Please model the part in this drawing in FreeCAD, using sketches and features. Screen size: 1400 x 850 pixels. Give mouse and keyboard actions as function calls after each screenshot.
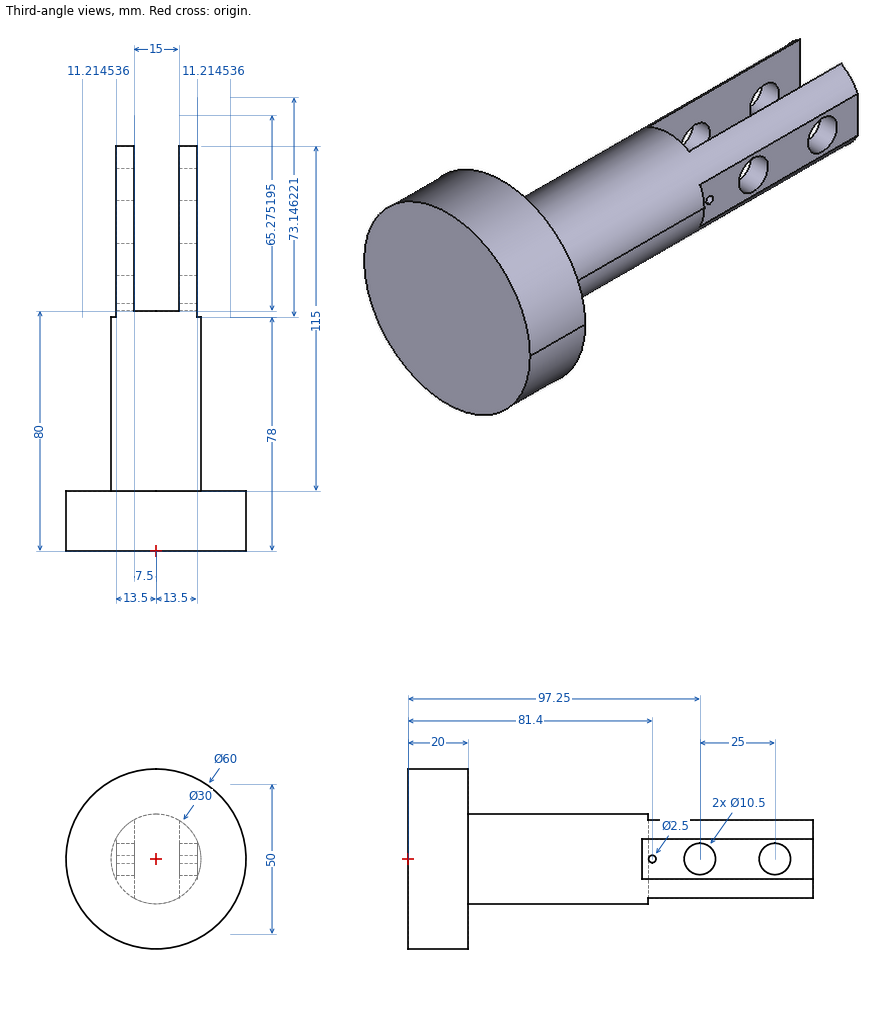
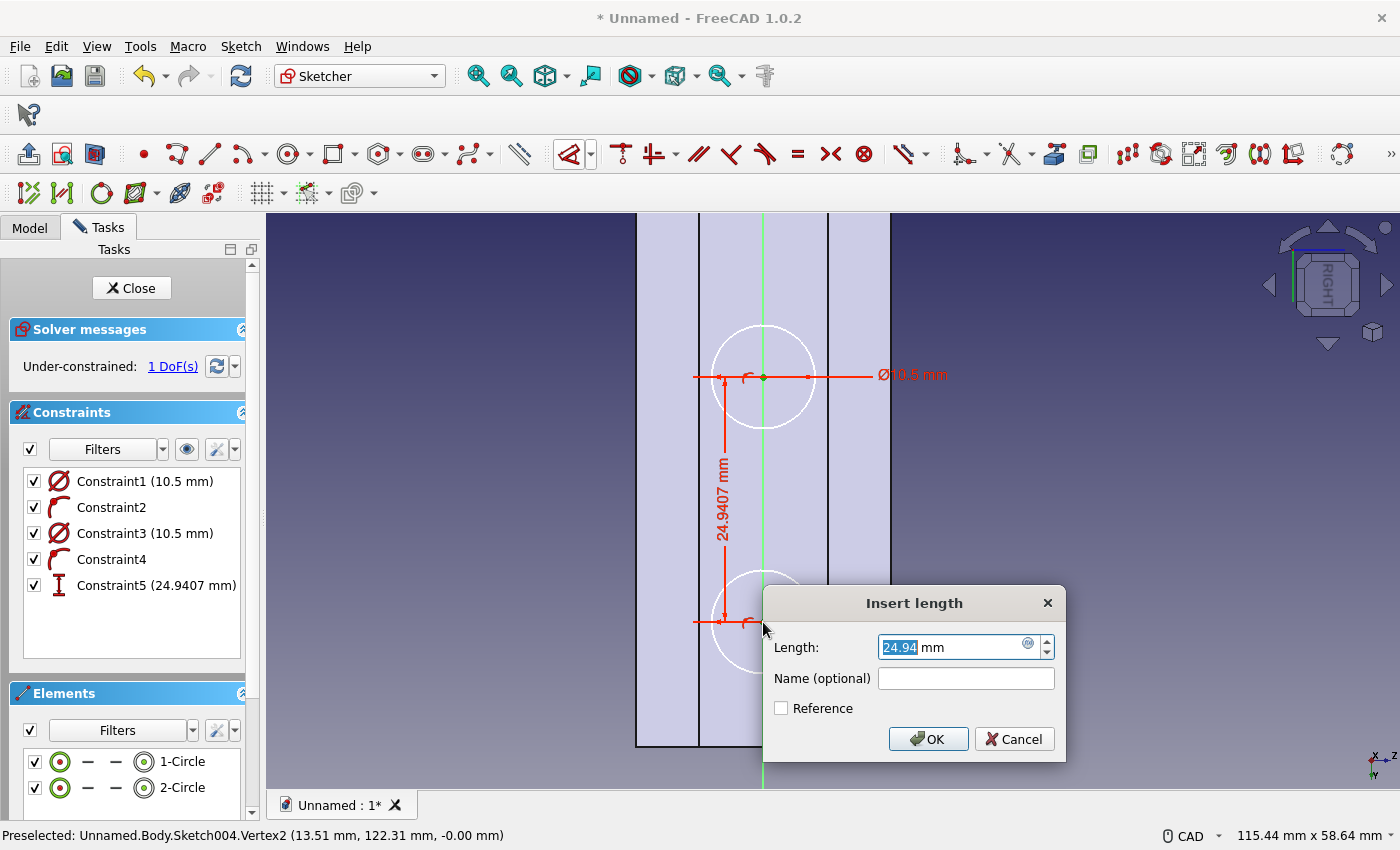
text(25)
key(Return)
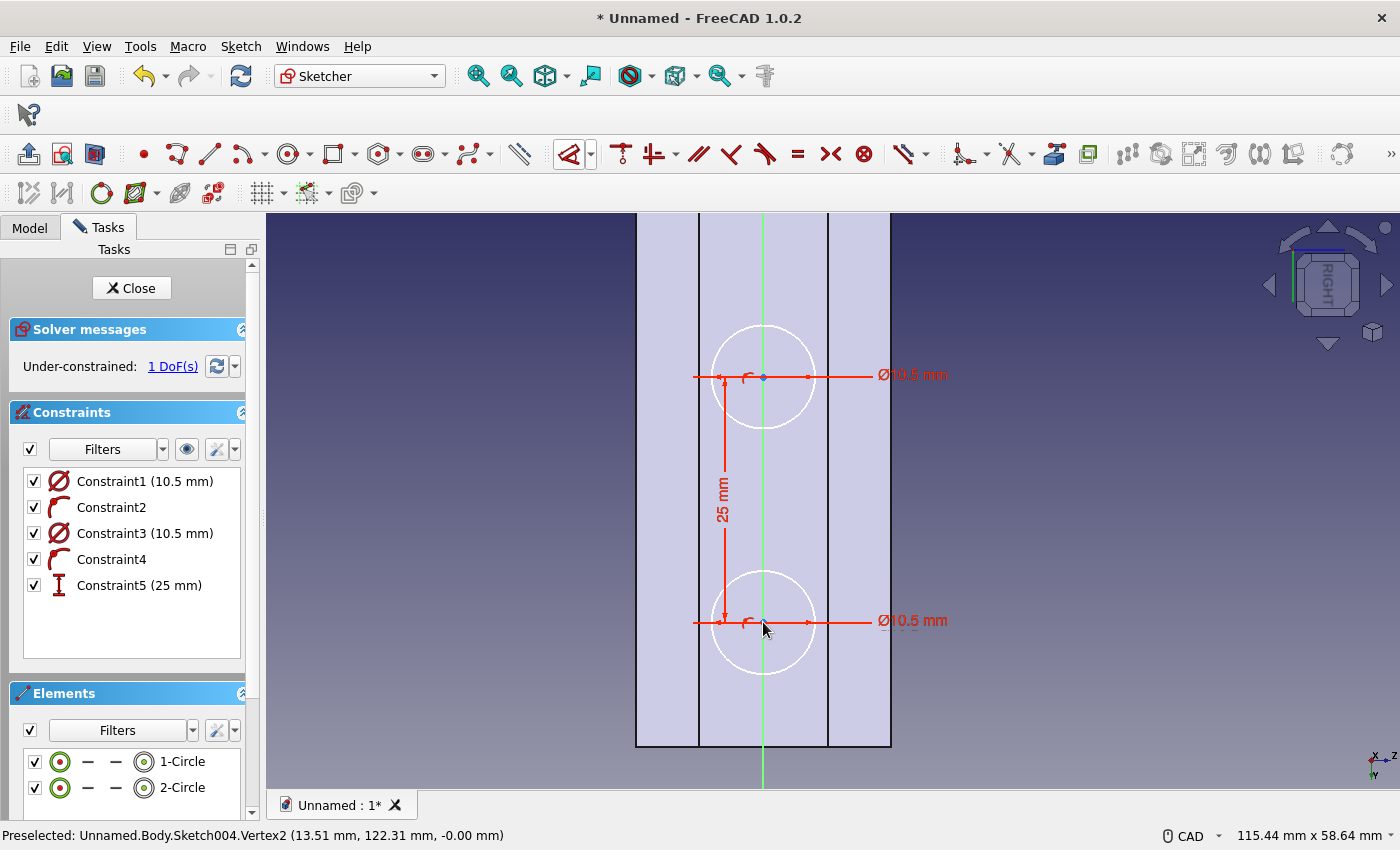
click(763, 377)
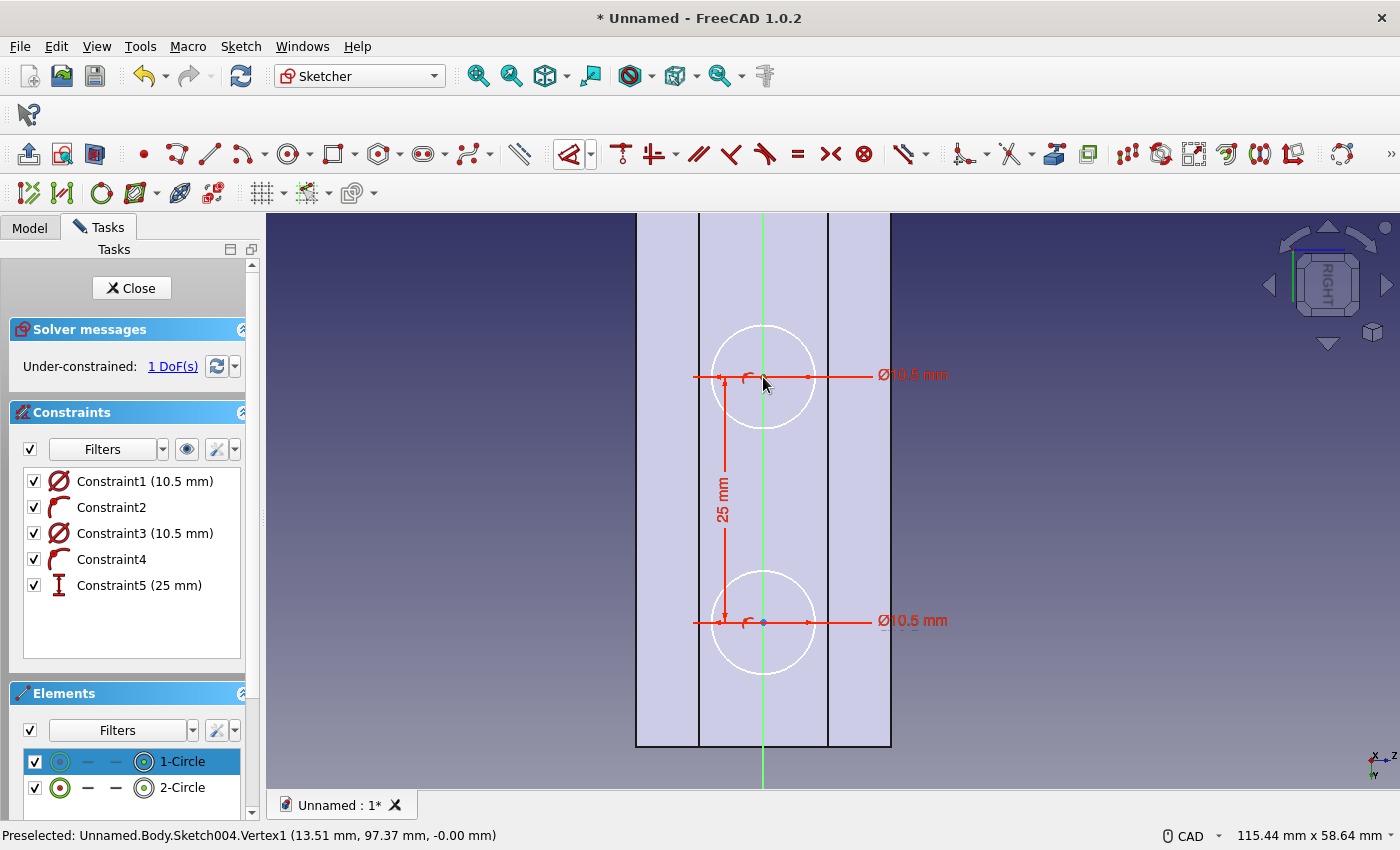
key(i)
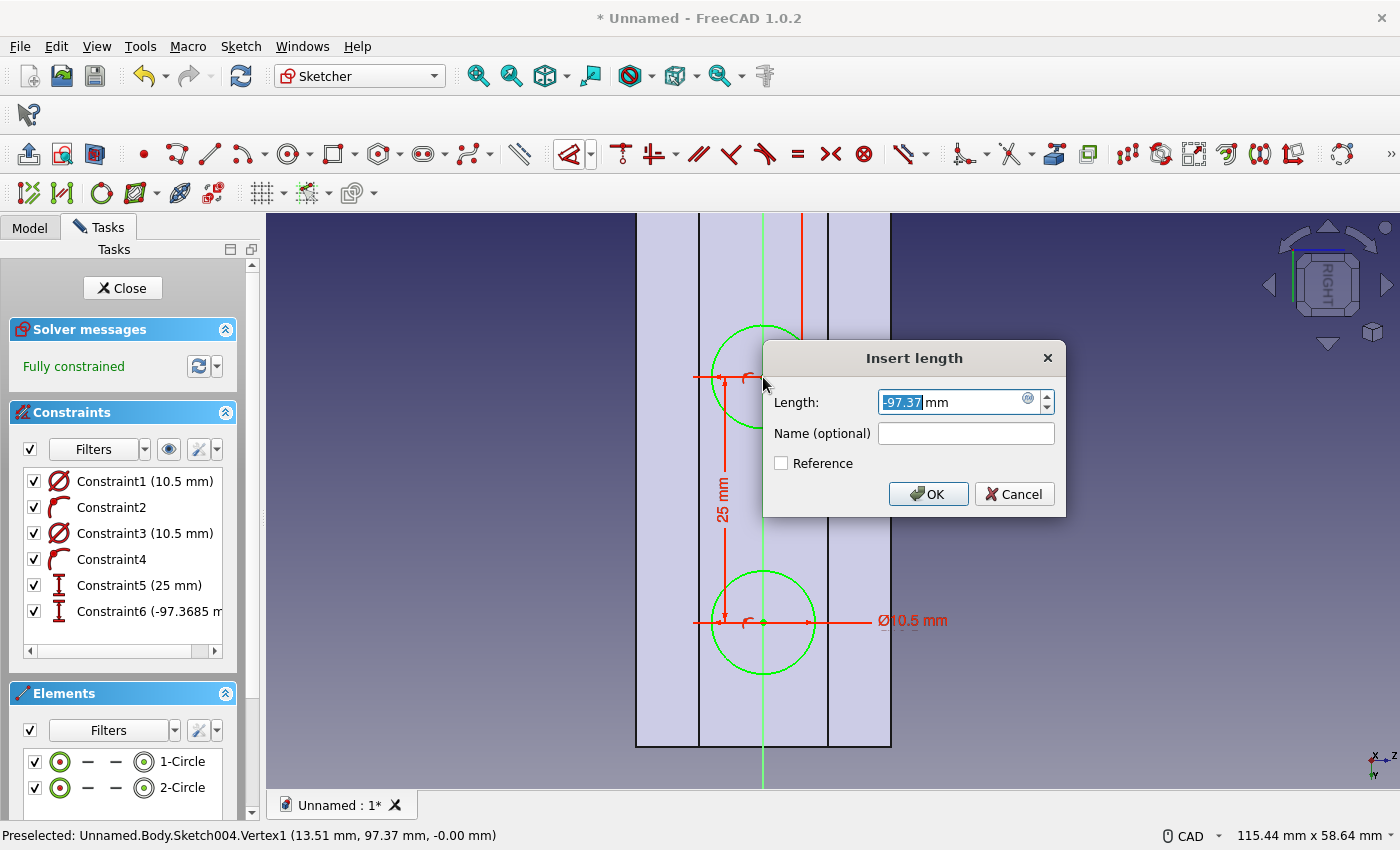
text(-97.25)
key(Return)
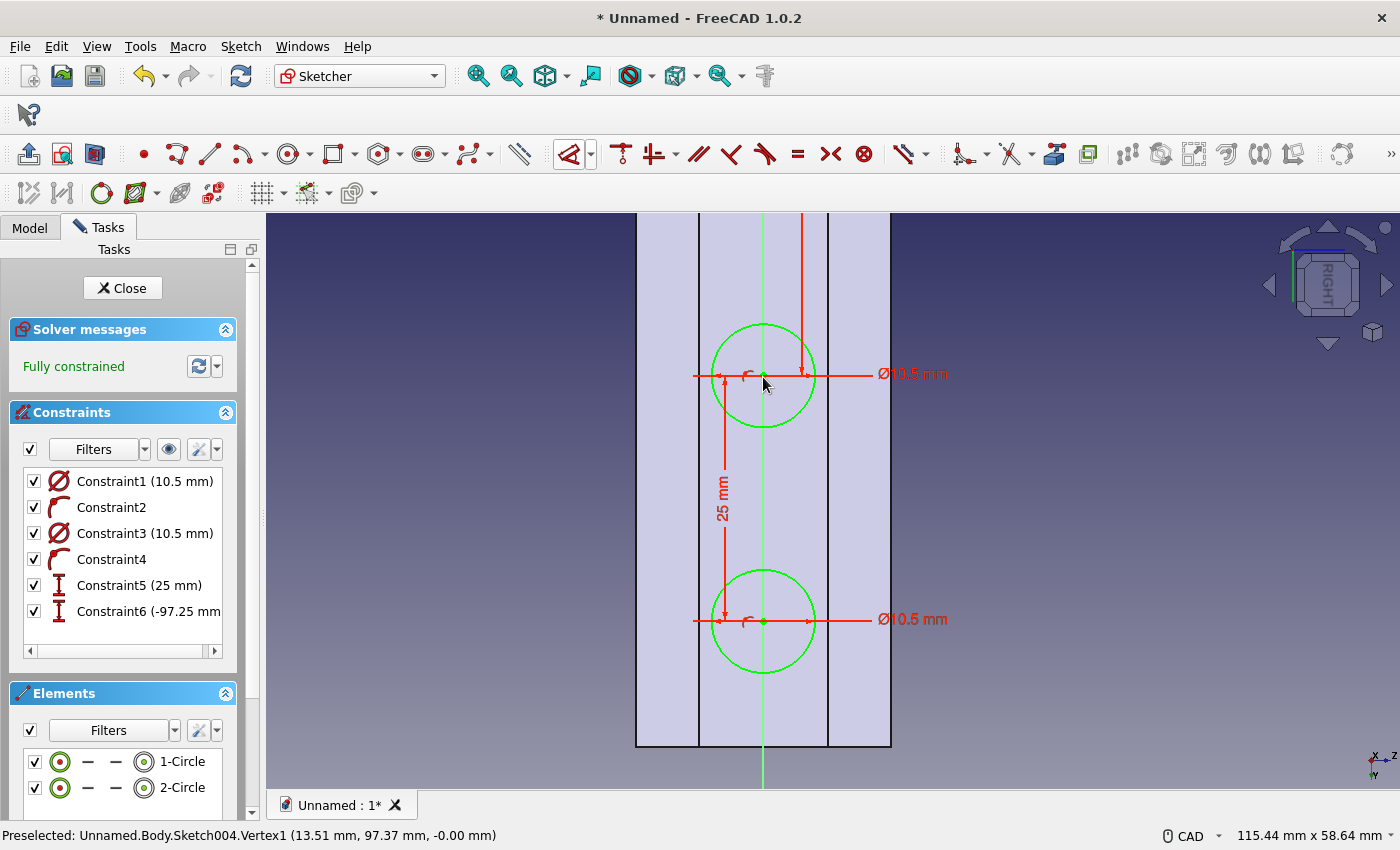
click(123, 288)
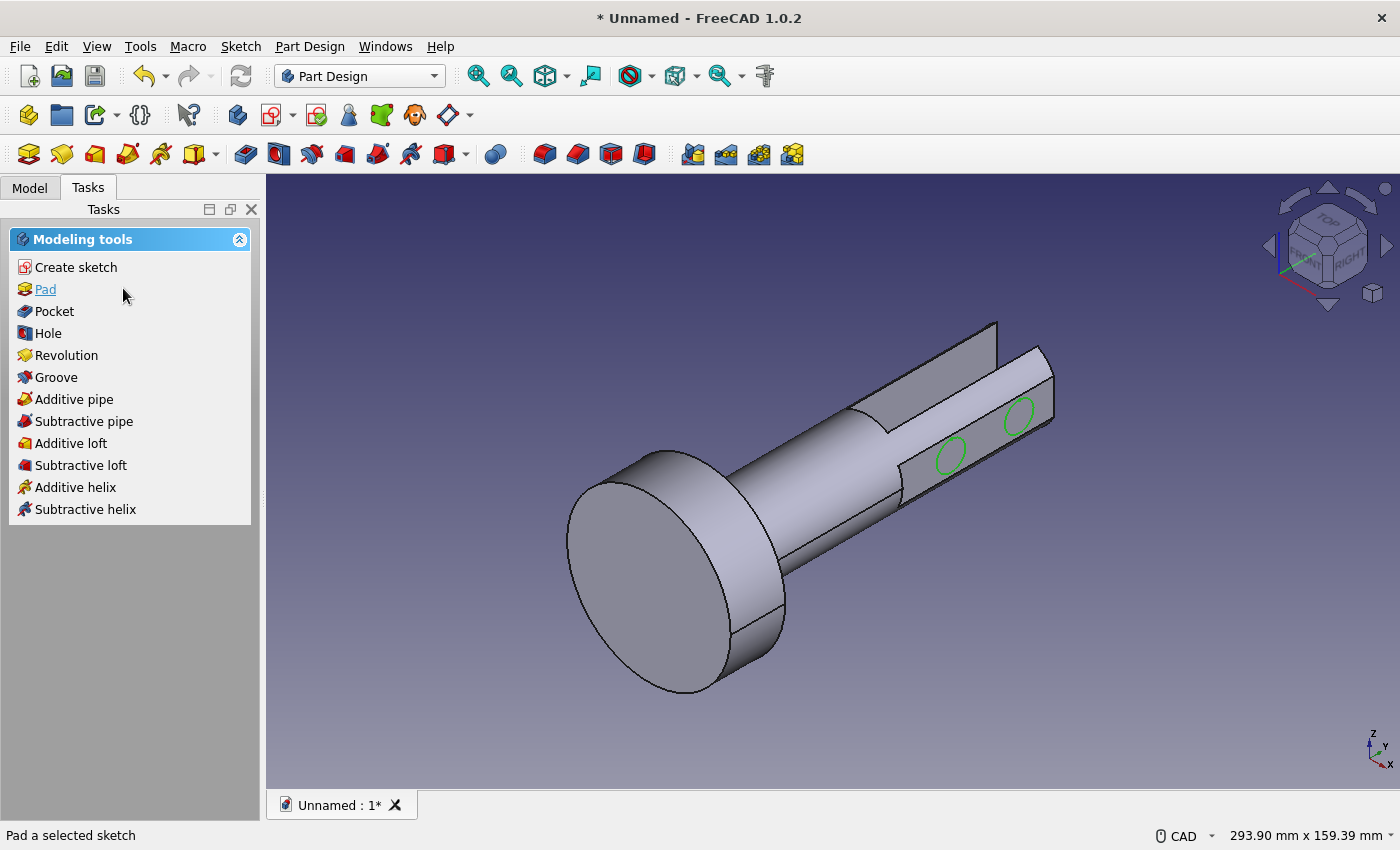
click(246, 154)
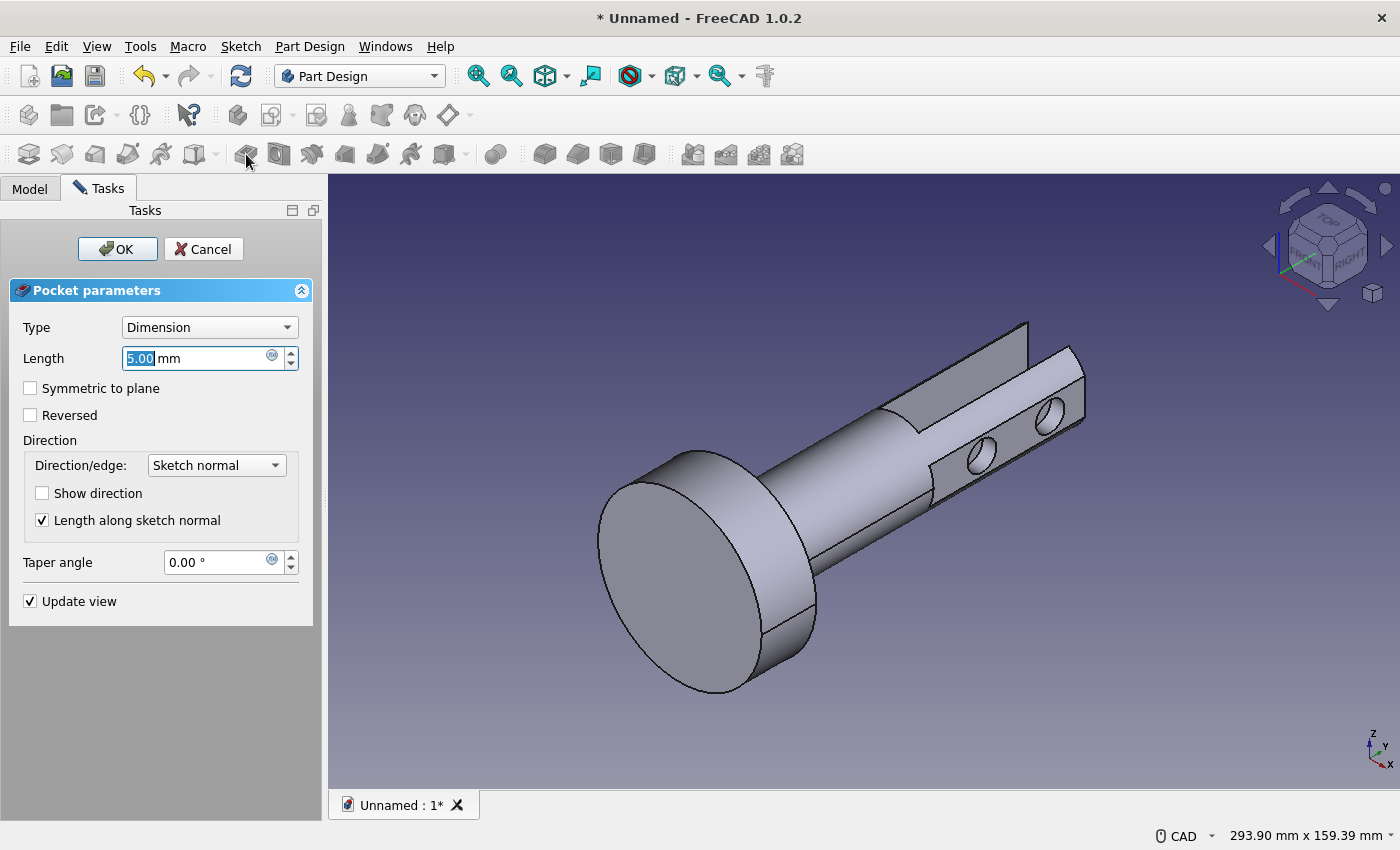
click(210, 328)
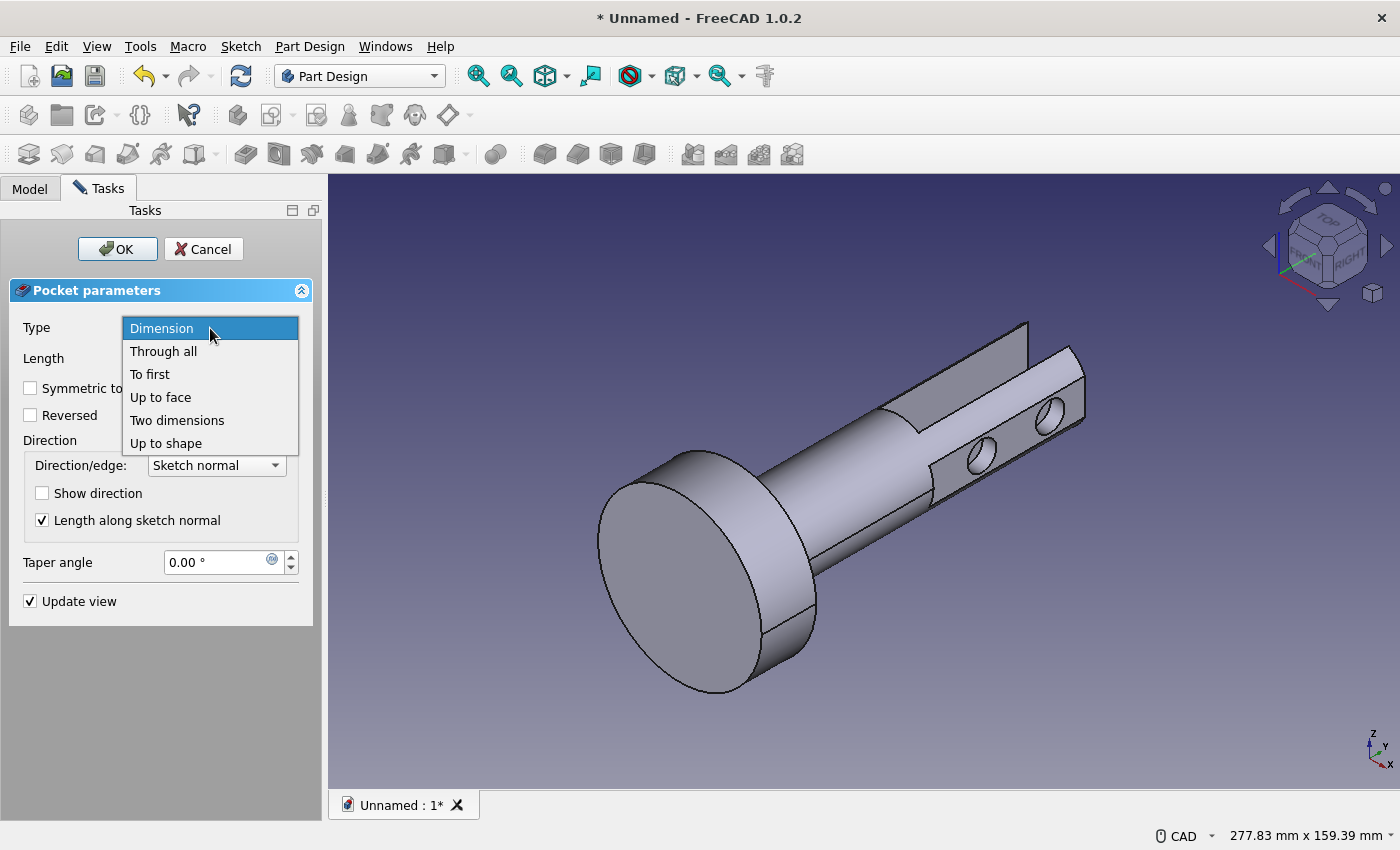
click(208, 352)